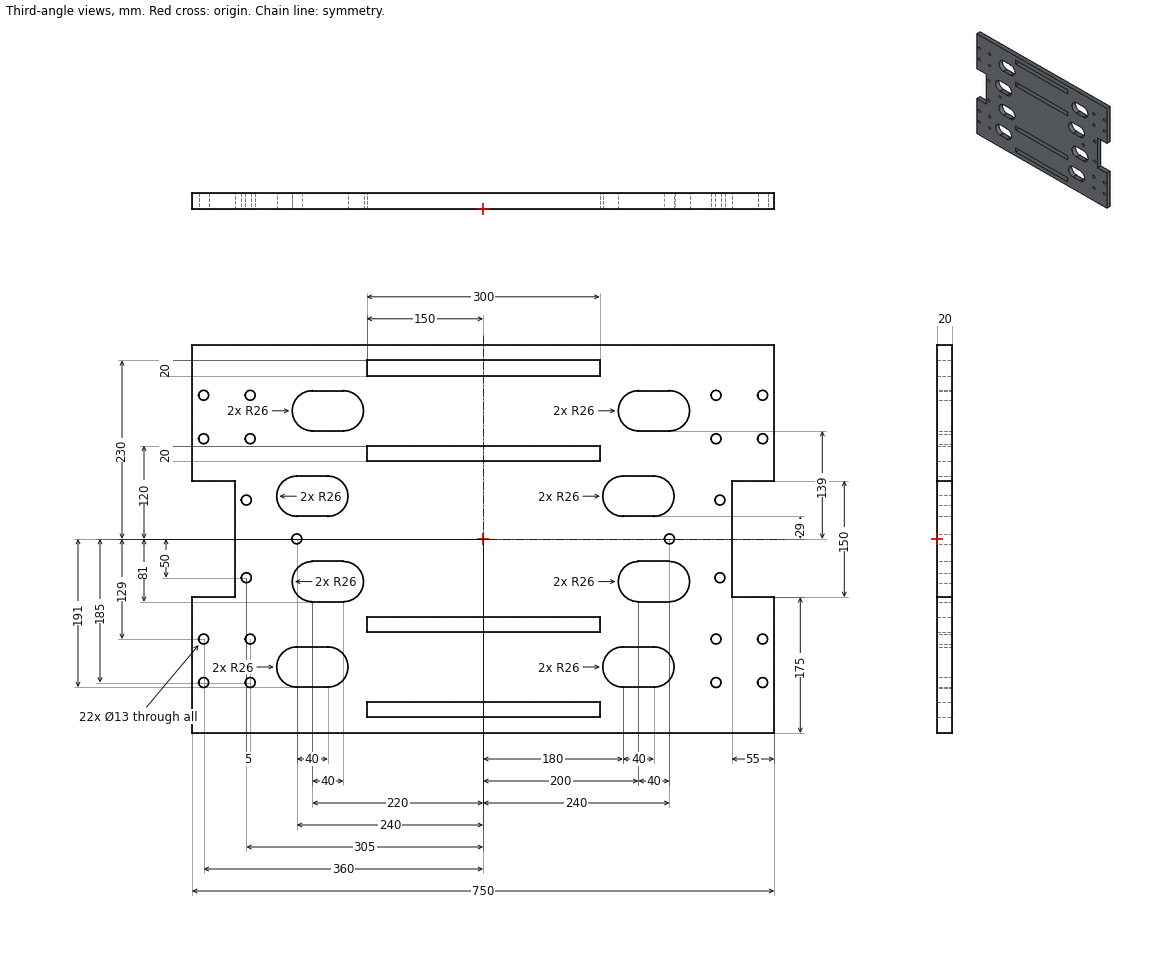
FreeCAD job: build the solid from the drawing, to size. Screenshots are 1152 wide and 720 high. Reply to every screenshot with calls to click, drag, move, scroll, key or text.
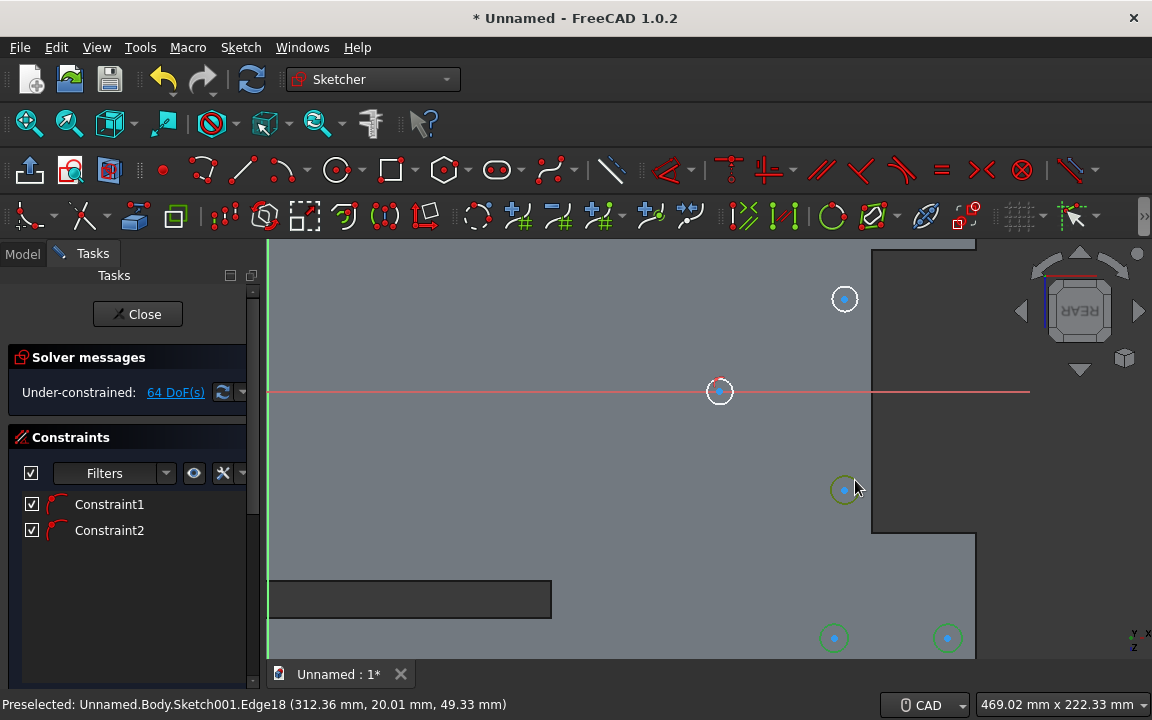
scroll(857, 482, down, 5)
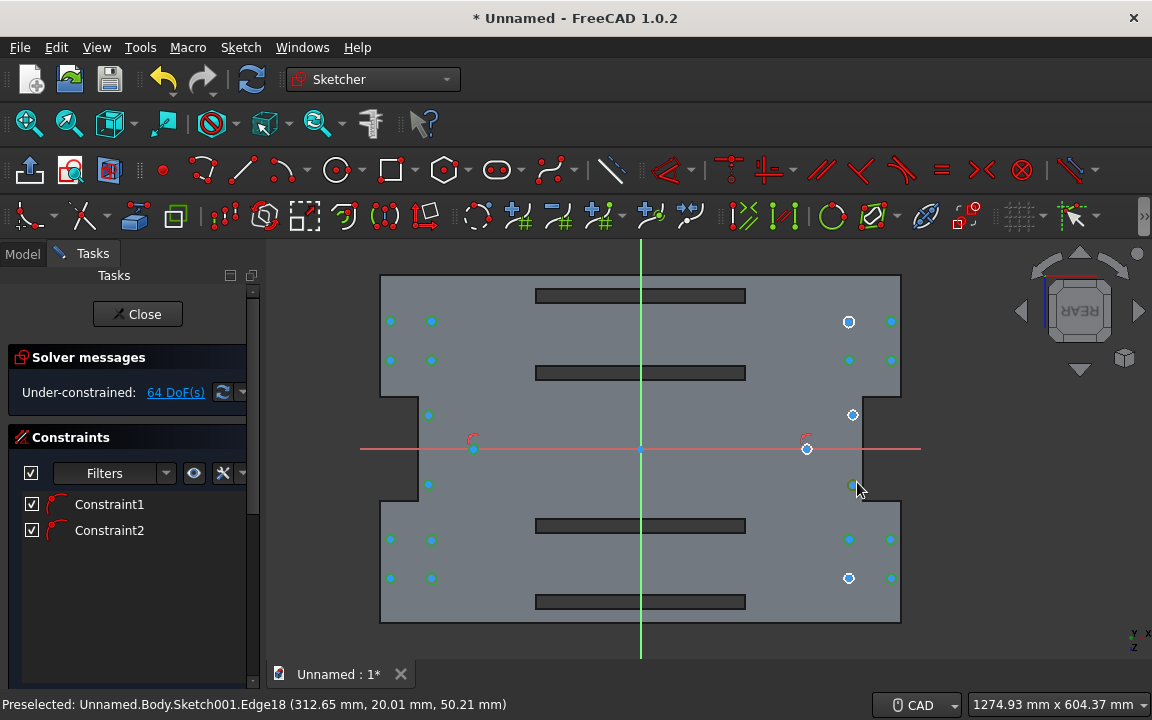
scroll(852, 575, up, 6)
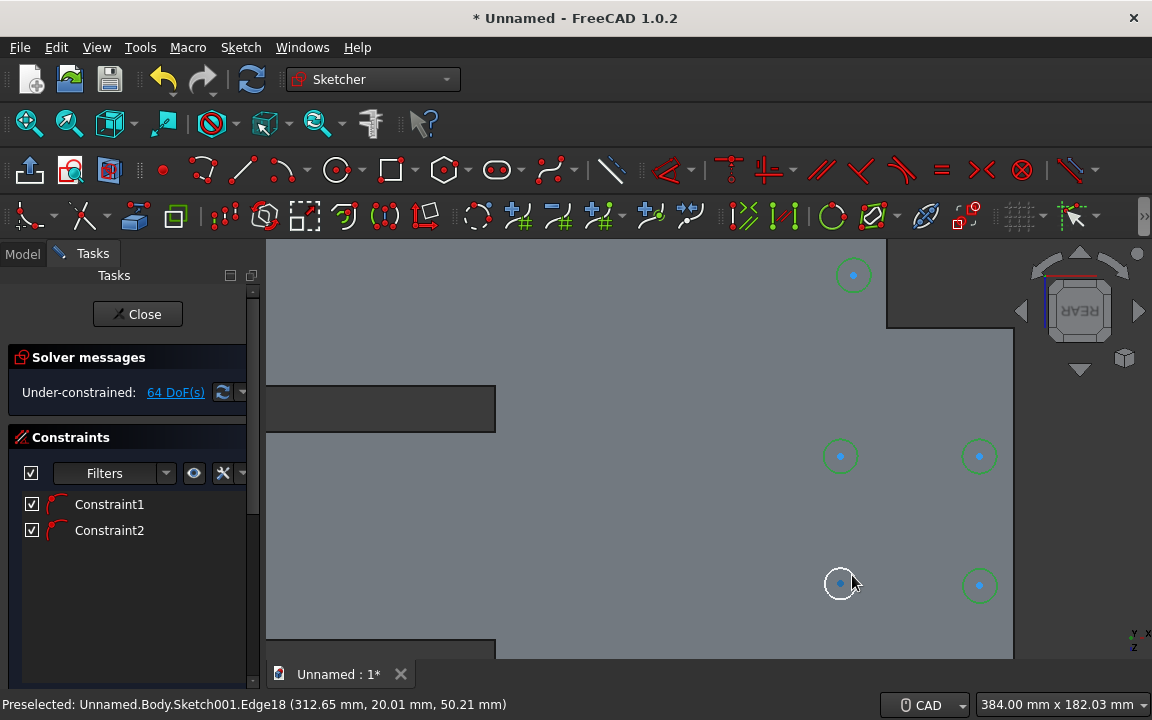
click(852, 573)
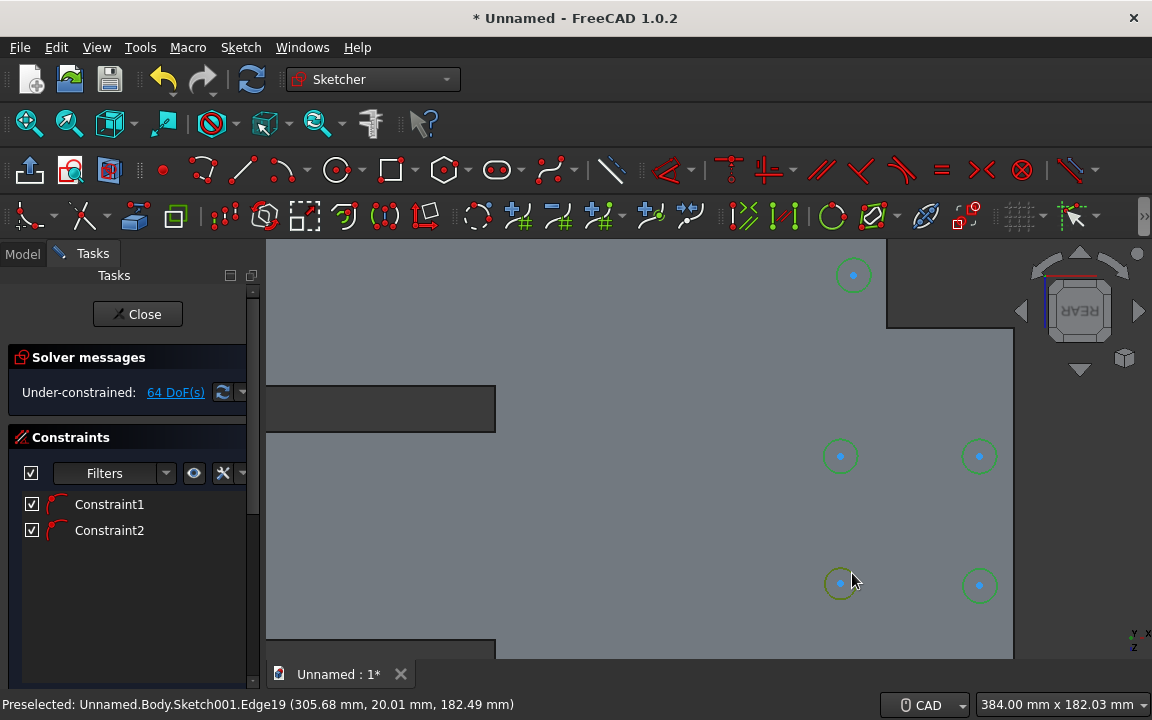
scroll(852, 576, down, 6)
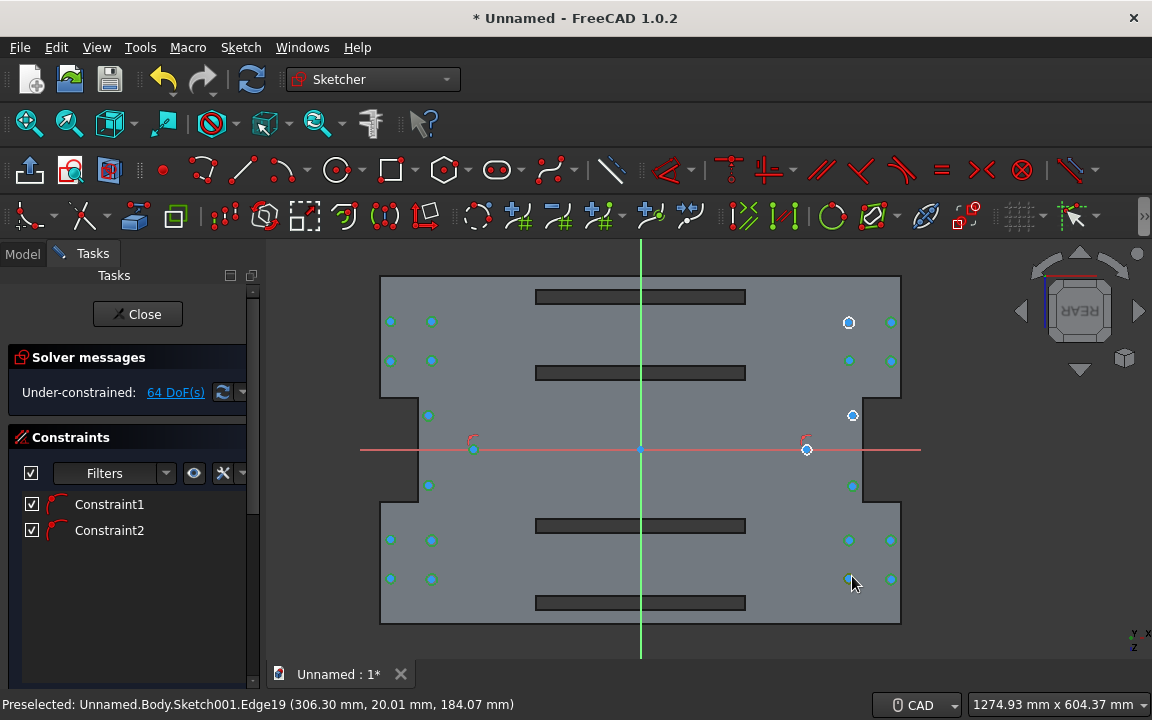
scroll(853, 319, up, 5)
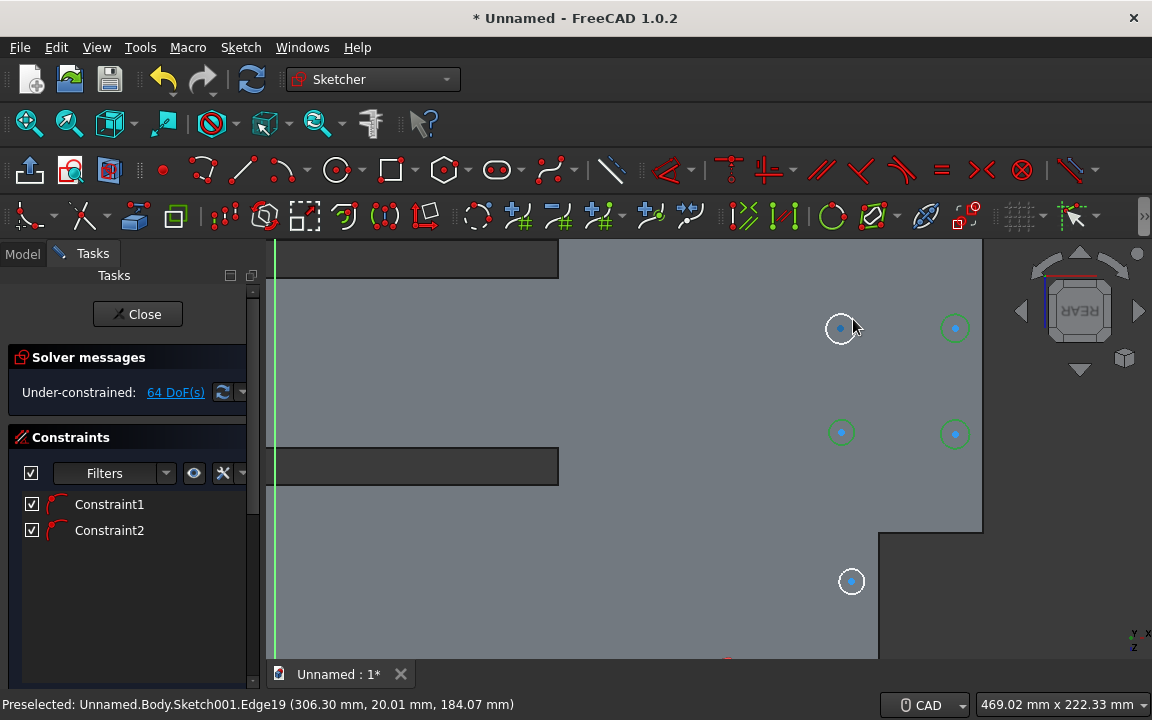
click(851, 318)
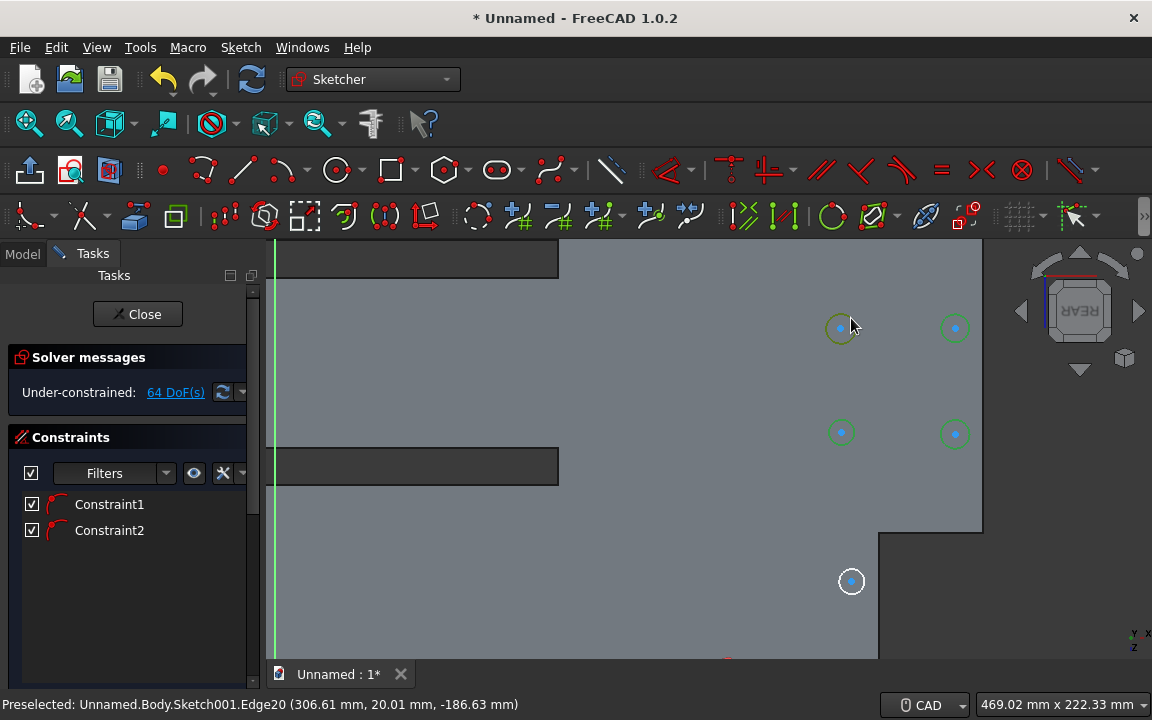
scroll(853, 318, down, 5)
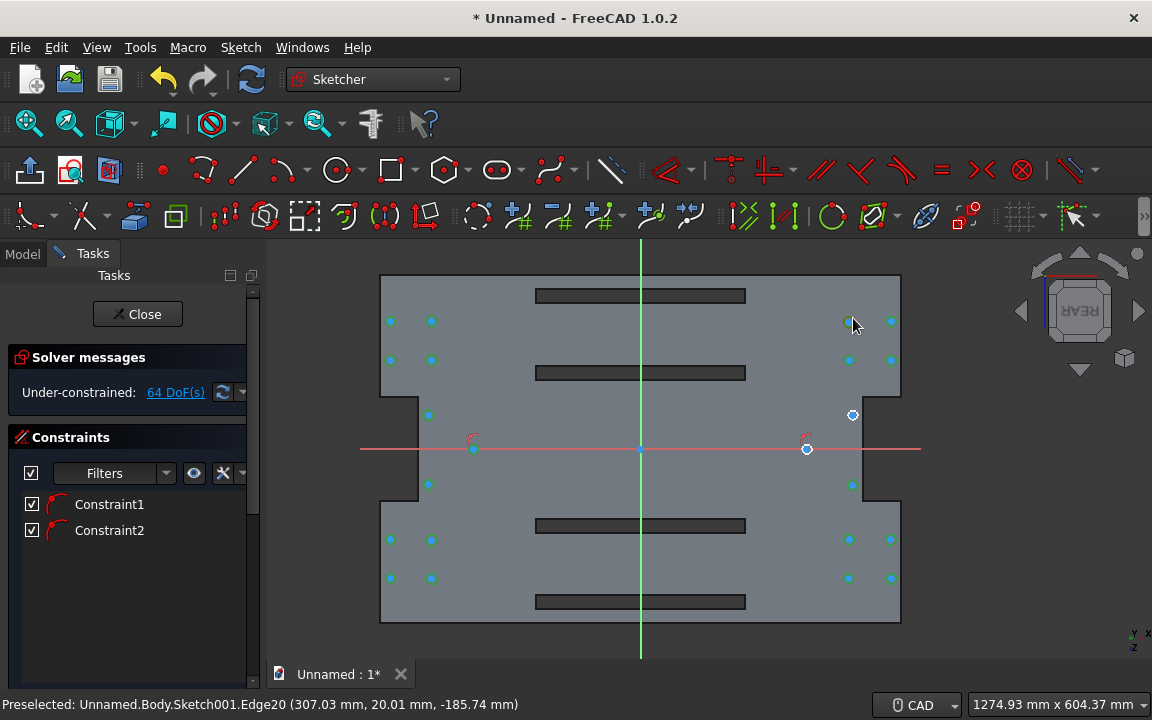
scroll(810, 446, up, 8)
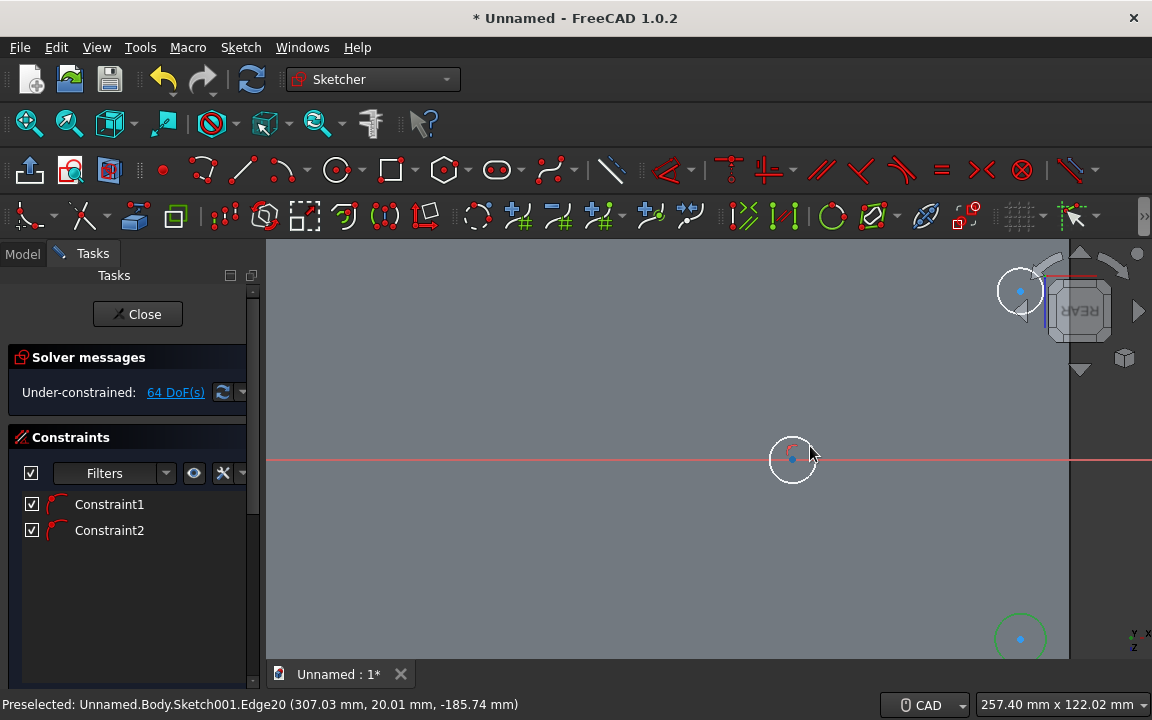
click(809, 444)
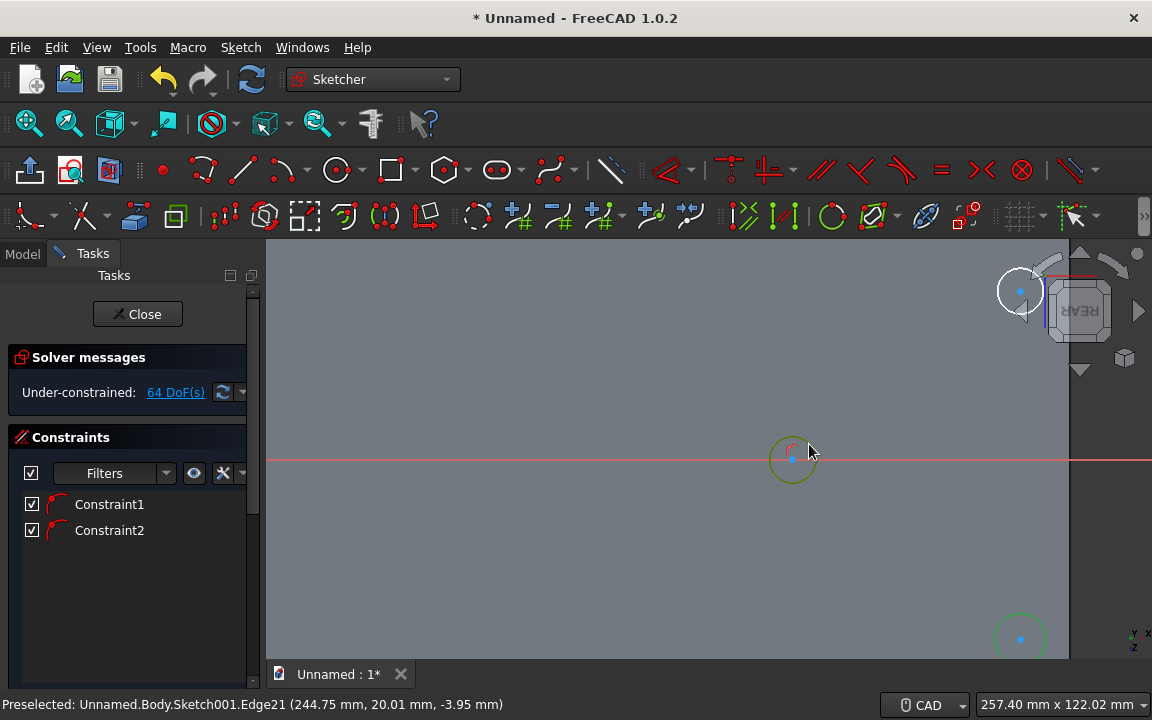
scroll(810, 446, down, 8)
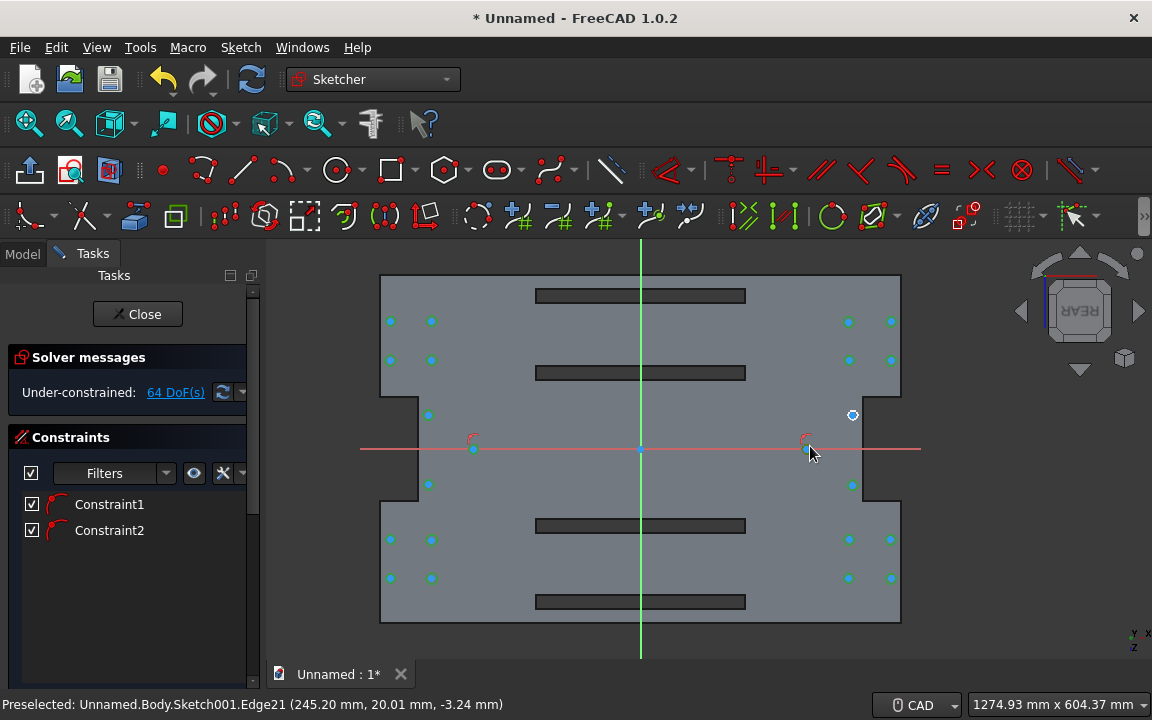
scroll(856, 412, up, 6)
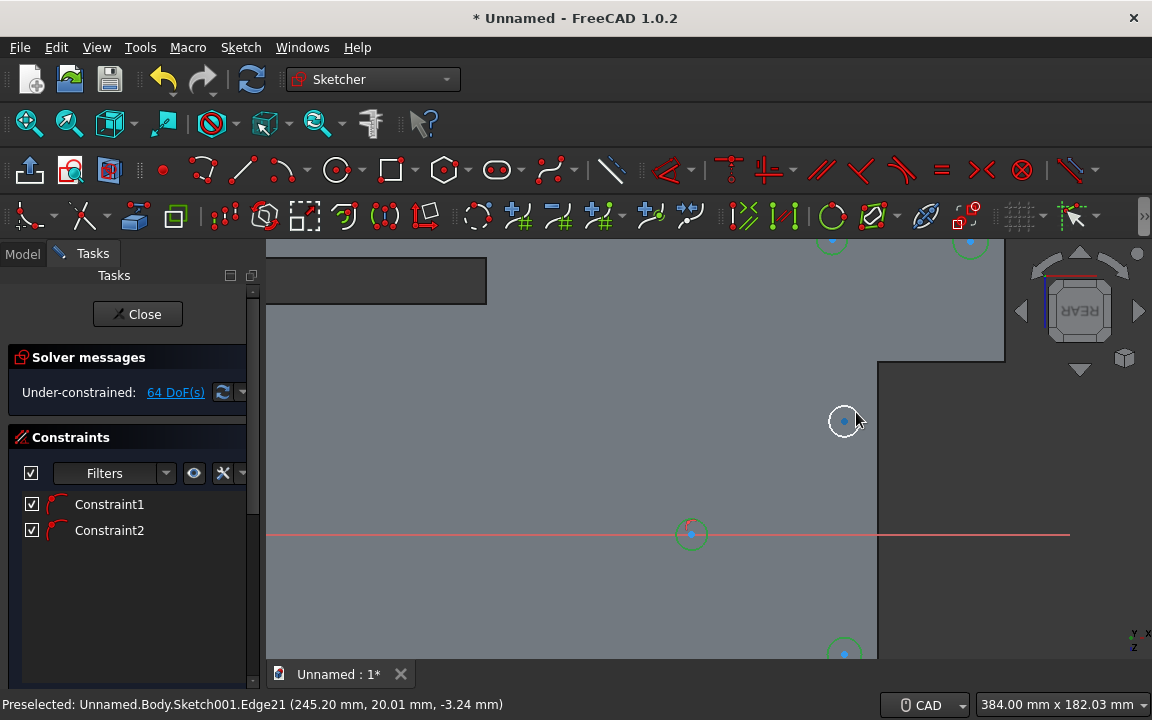
click(855, 411)